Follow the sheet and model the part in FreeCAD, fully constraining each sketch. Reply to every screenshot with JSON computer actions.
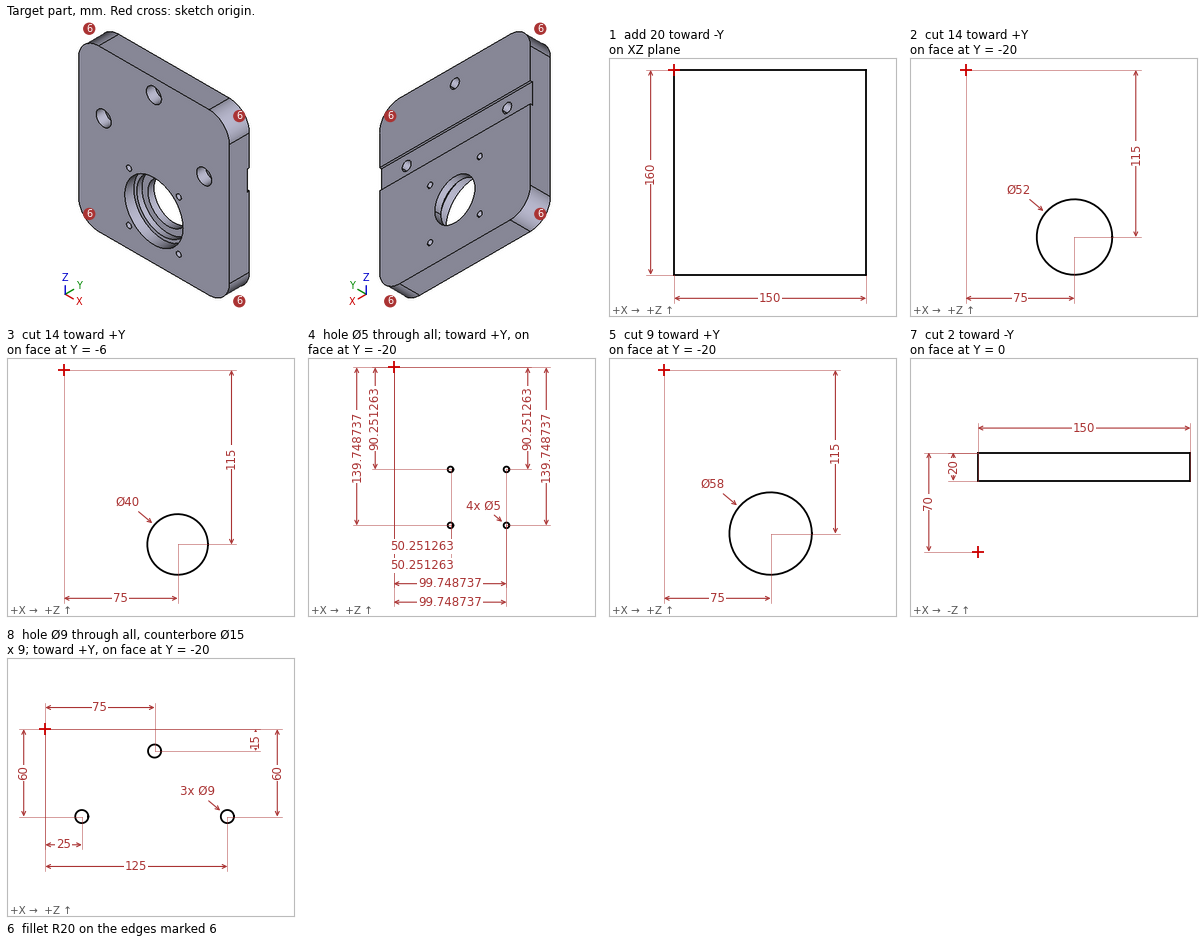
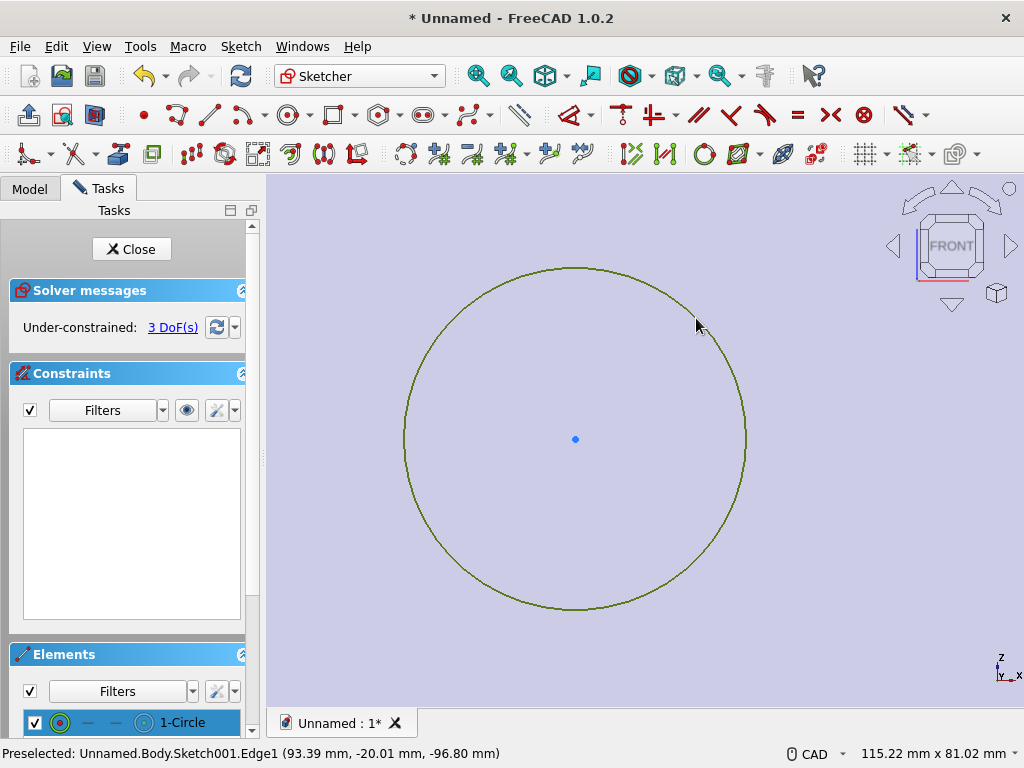
{"action": "left_click", "coordinate": [590, 116]}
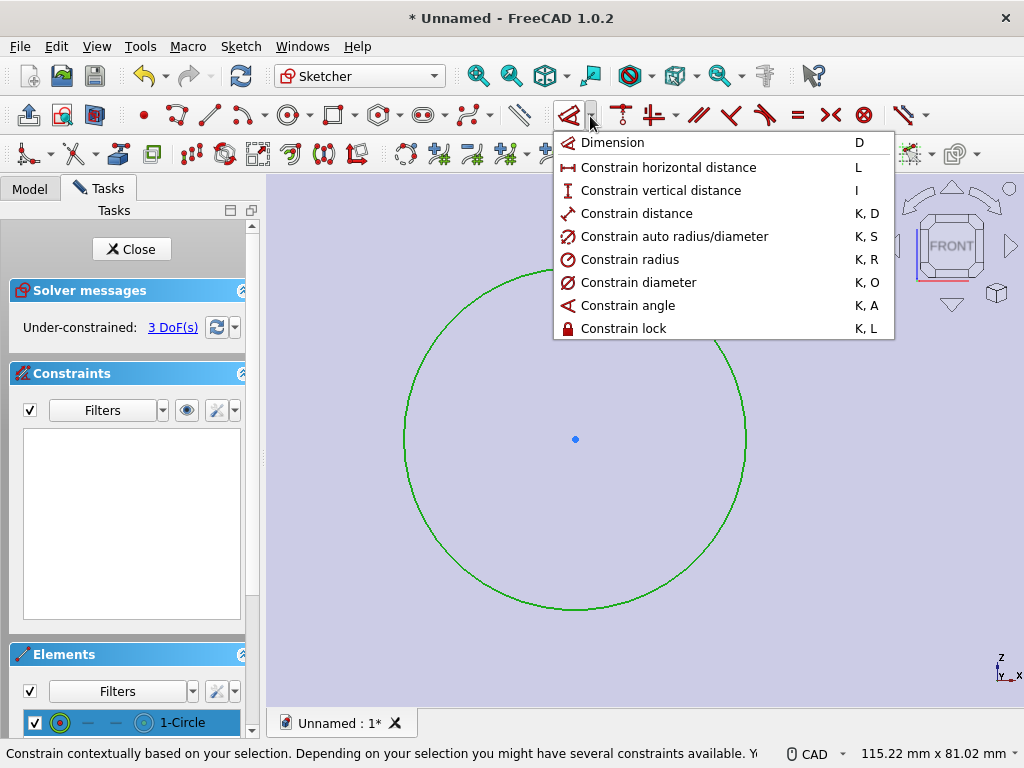
{"action": "left_click", "coordinate": [724, 282]}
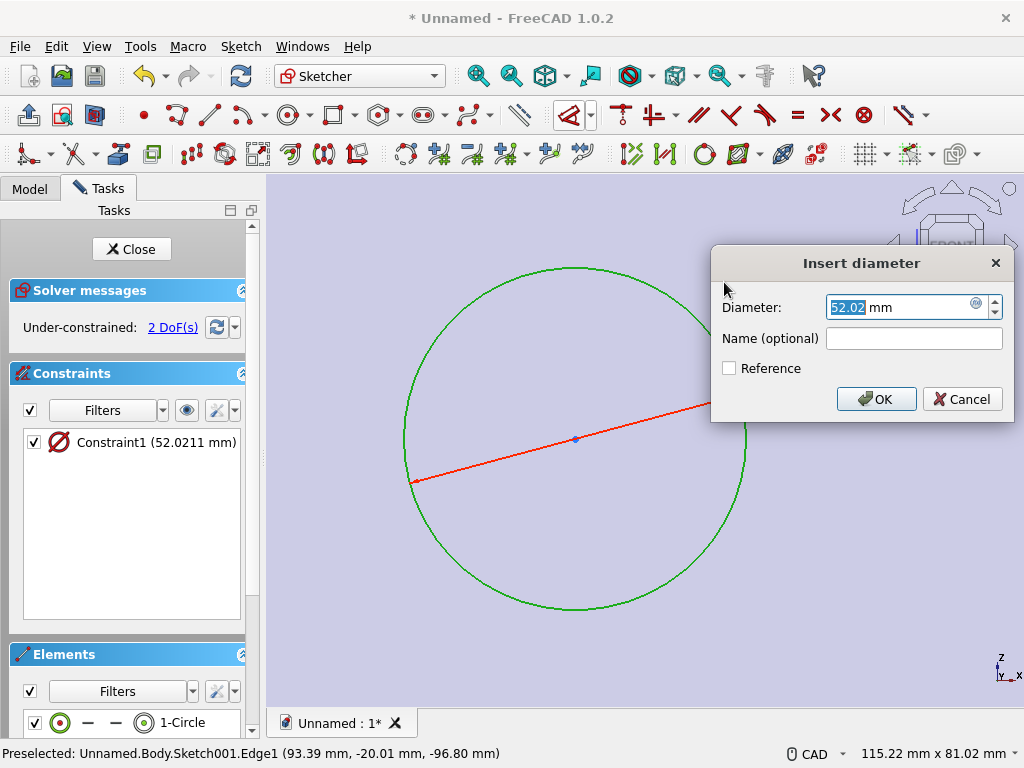
{"action": "type", "text": "52"}
{"action": "key", "text": "Return"}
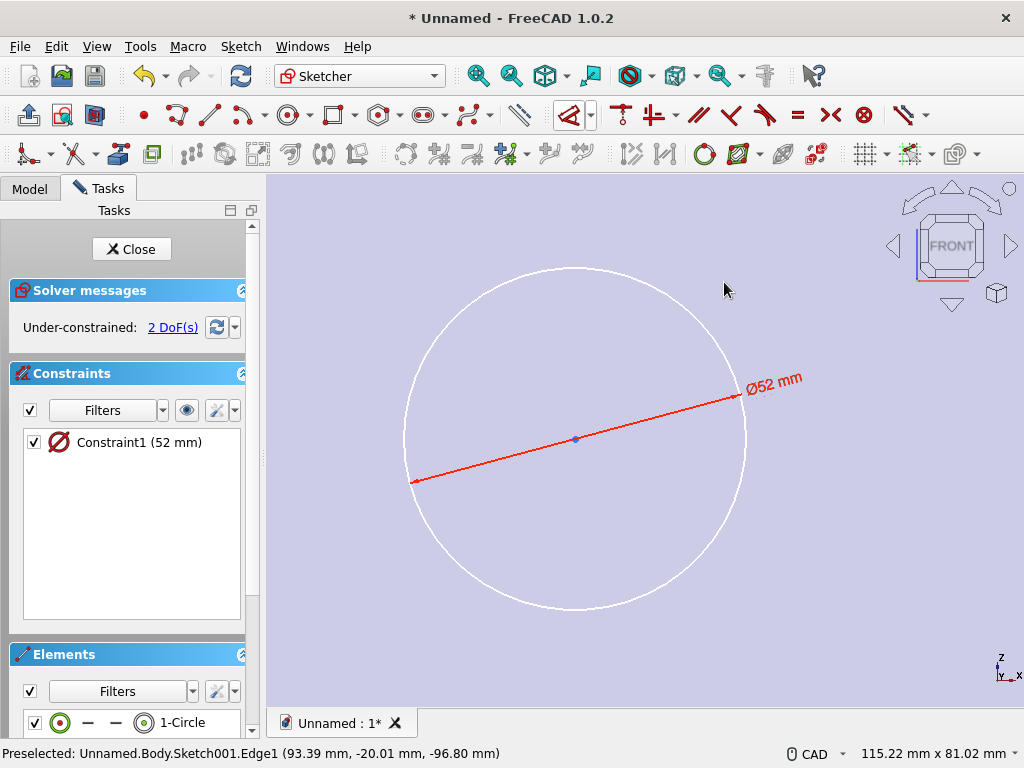
{"action": "left_click", "coordinate": [575, 439]}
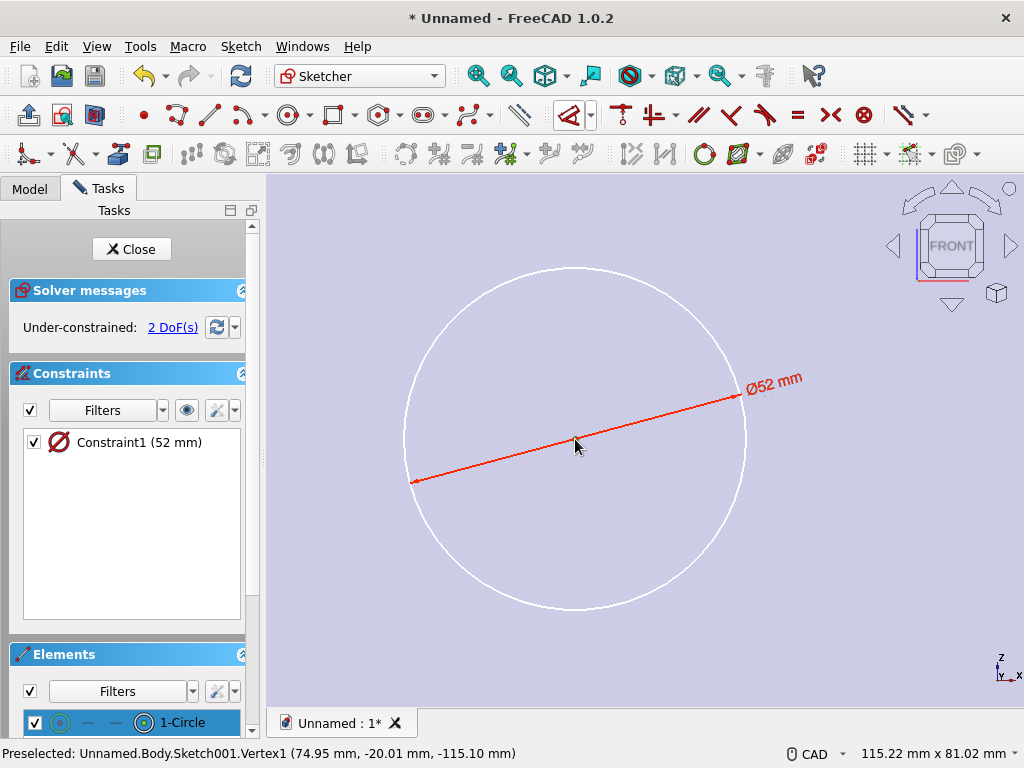
{"action": "key", "text": "l"}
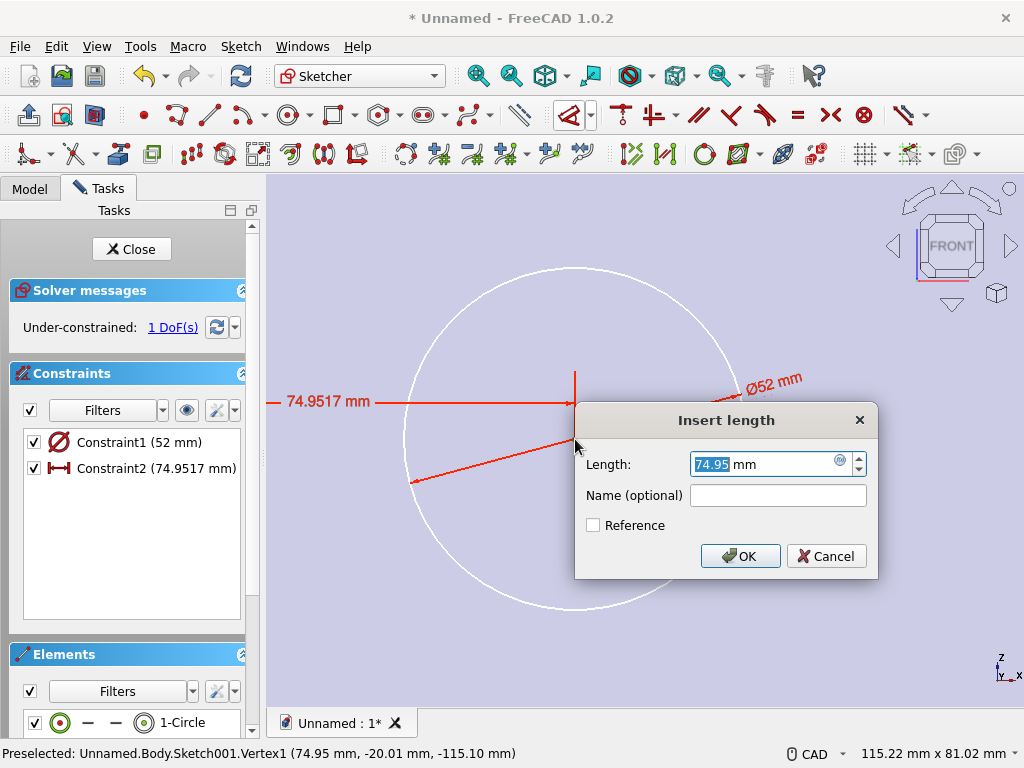
{"action": "type", "text": "75"}
{"action": "key", "text": "Return"}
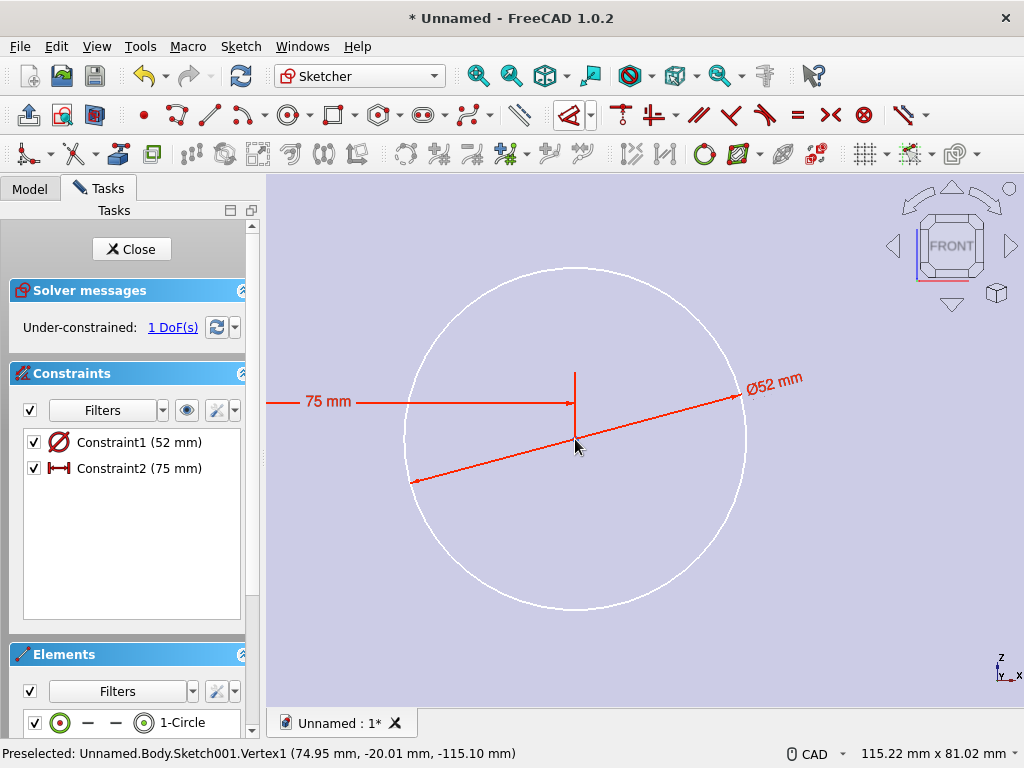
{"action": "left_click", "coordinate": [575, 439]}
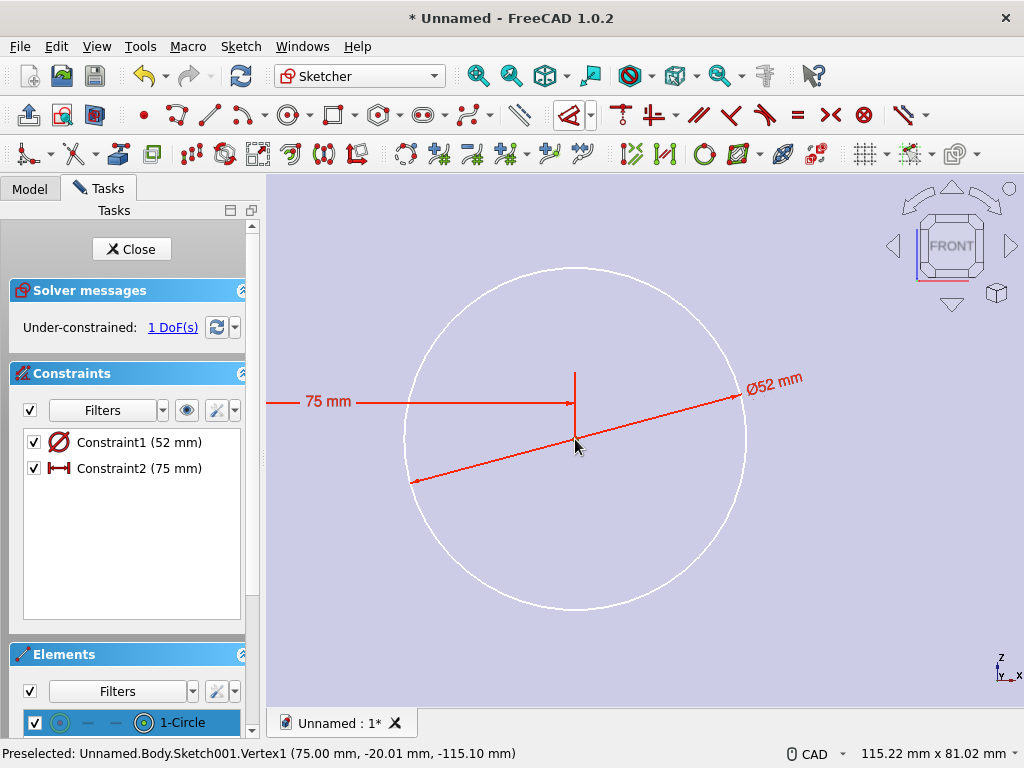
{"action": "left_click", "coordinate": [590, 116]}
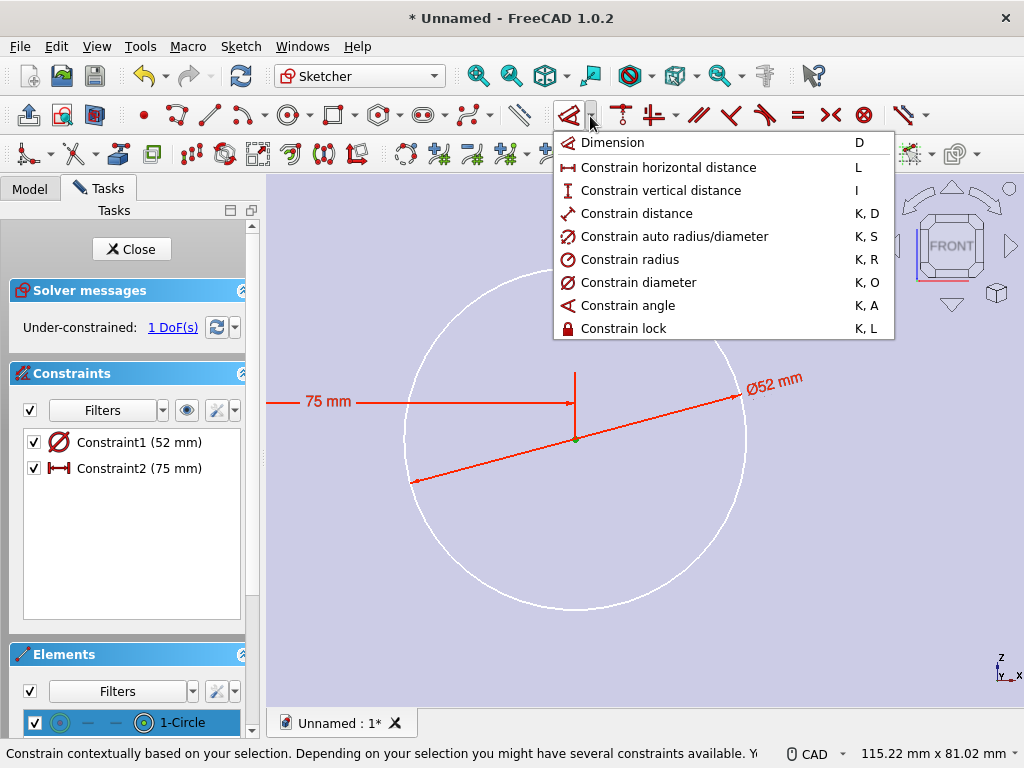
{"action": "left_click", "coordinate": [724, 190]}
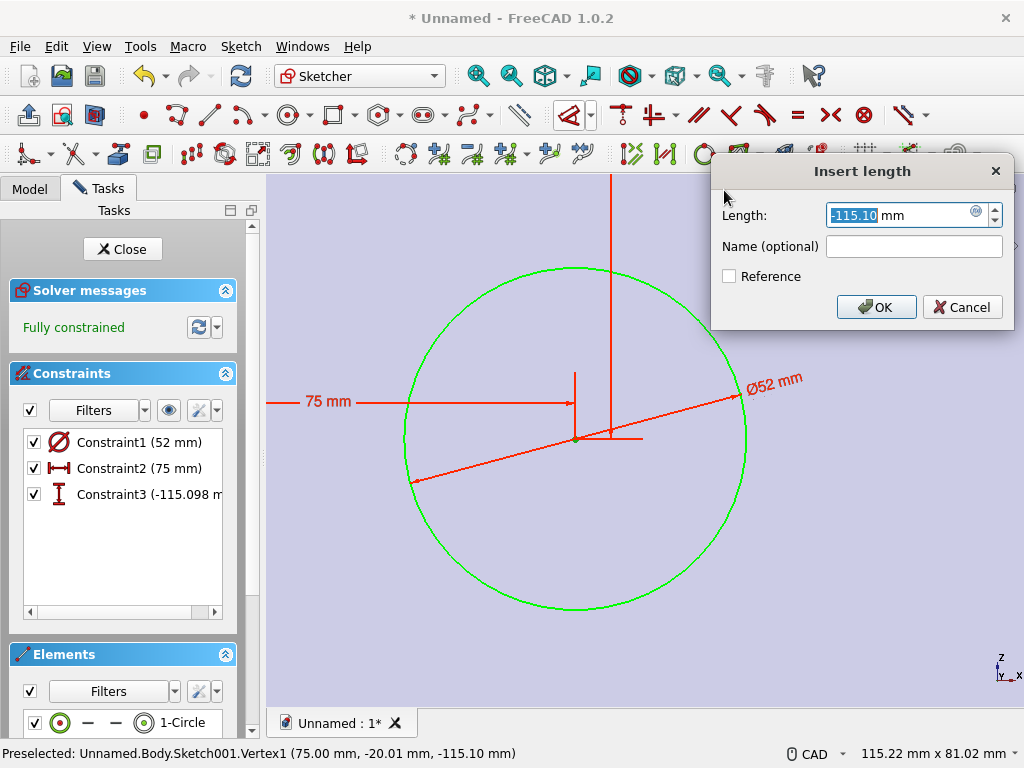
{"action": "type", "text": "-115"}
{"action": "key", "text": "Return"}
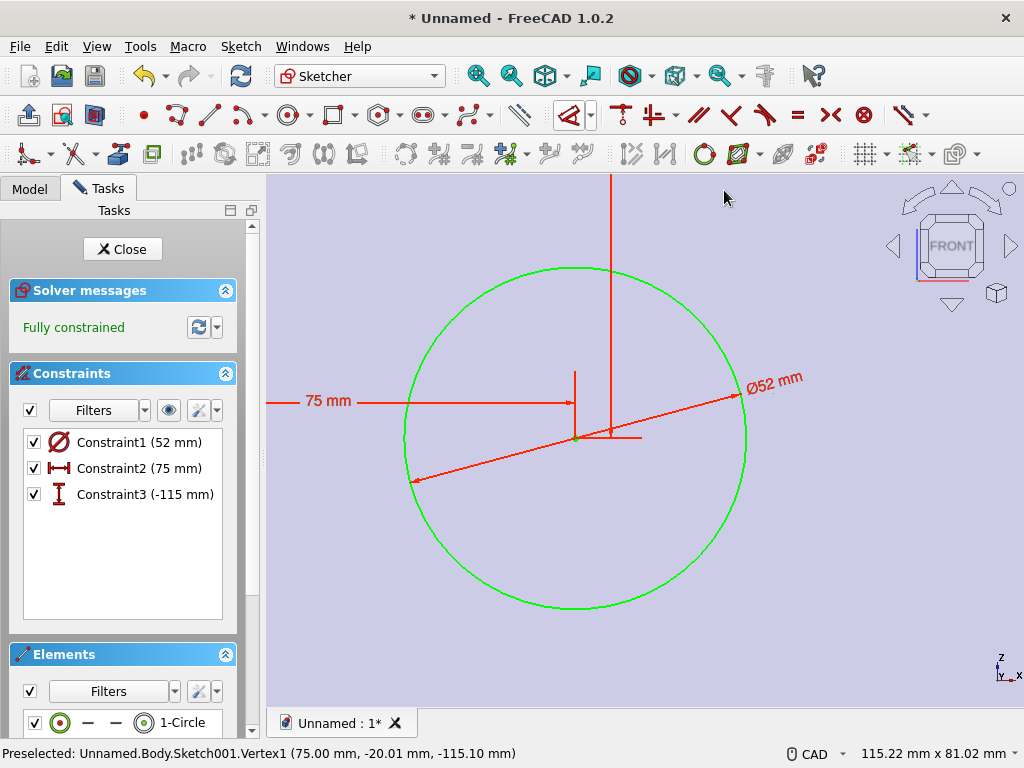
{"action": "left_click", "coordinate": [123, 249]}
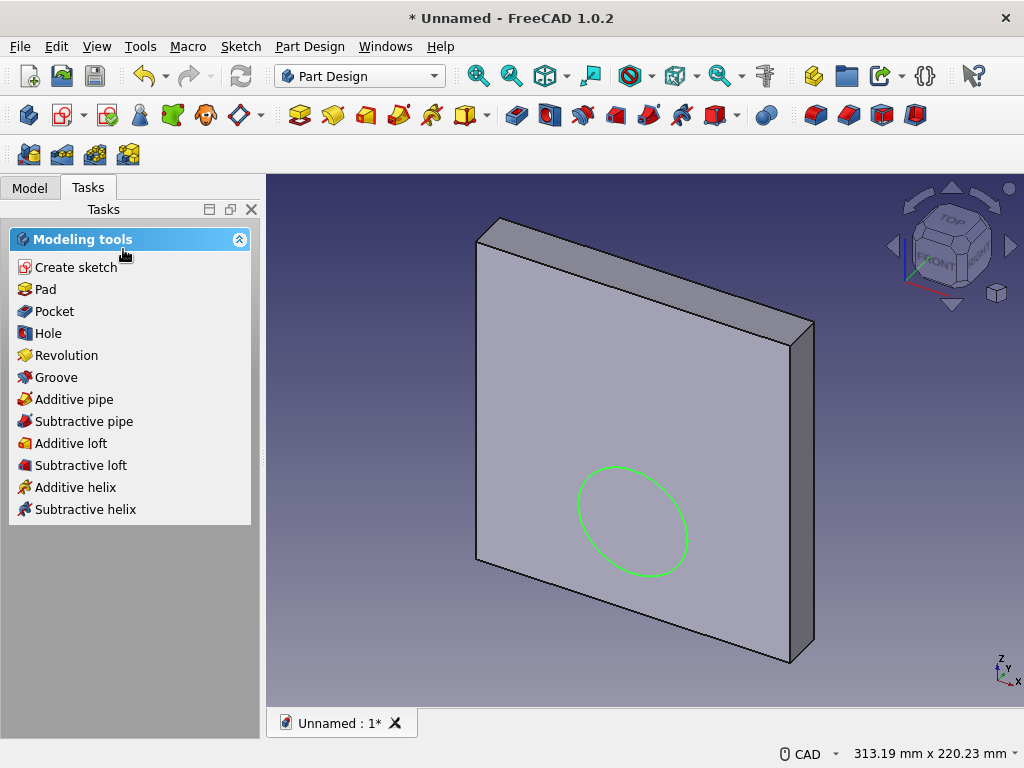
{"action": "left_click", "coordinate": [517, 116]}